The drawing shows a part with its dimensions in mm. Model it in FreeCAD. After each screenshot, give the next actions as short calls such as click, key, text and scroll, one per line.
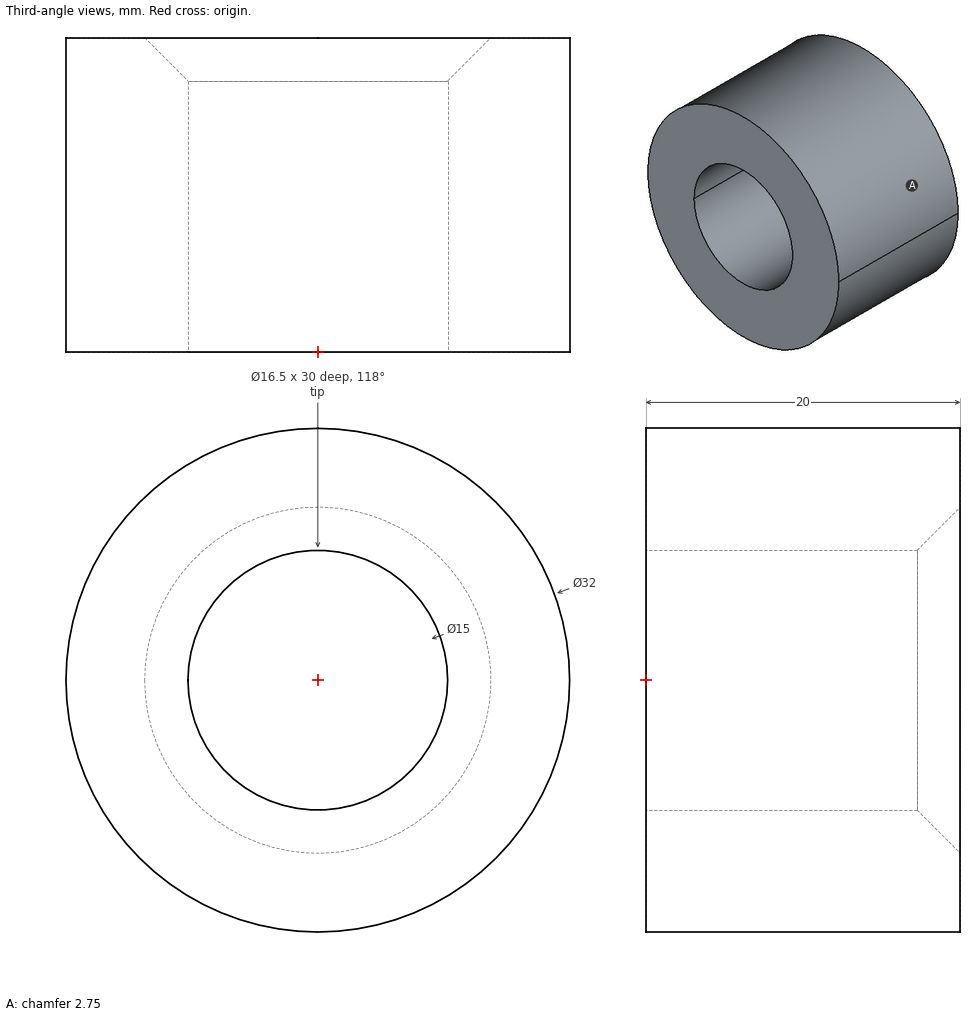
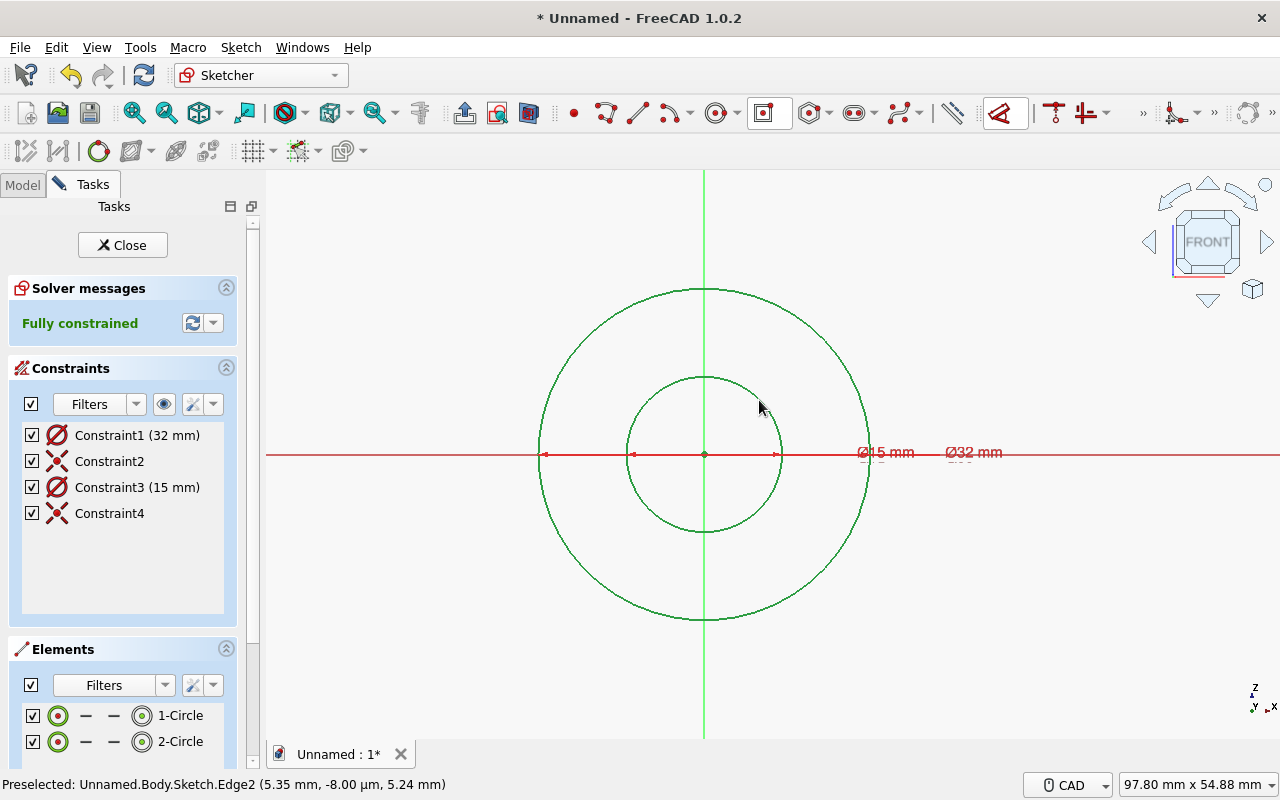
click(123, 245)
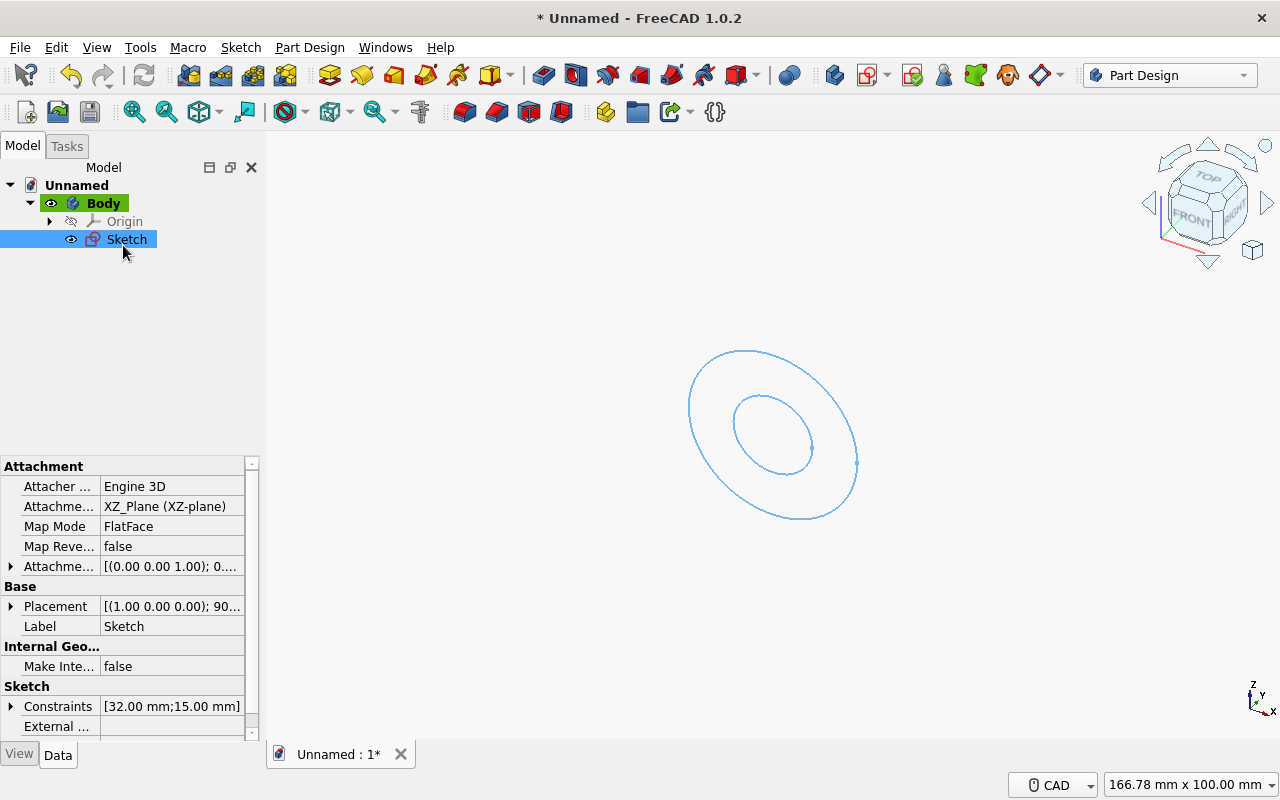
click(330, 76)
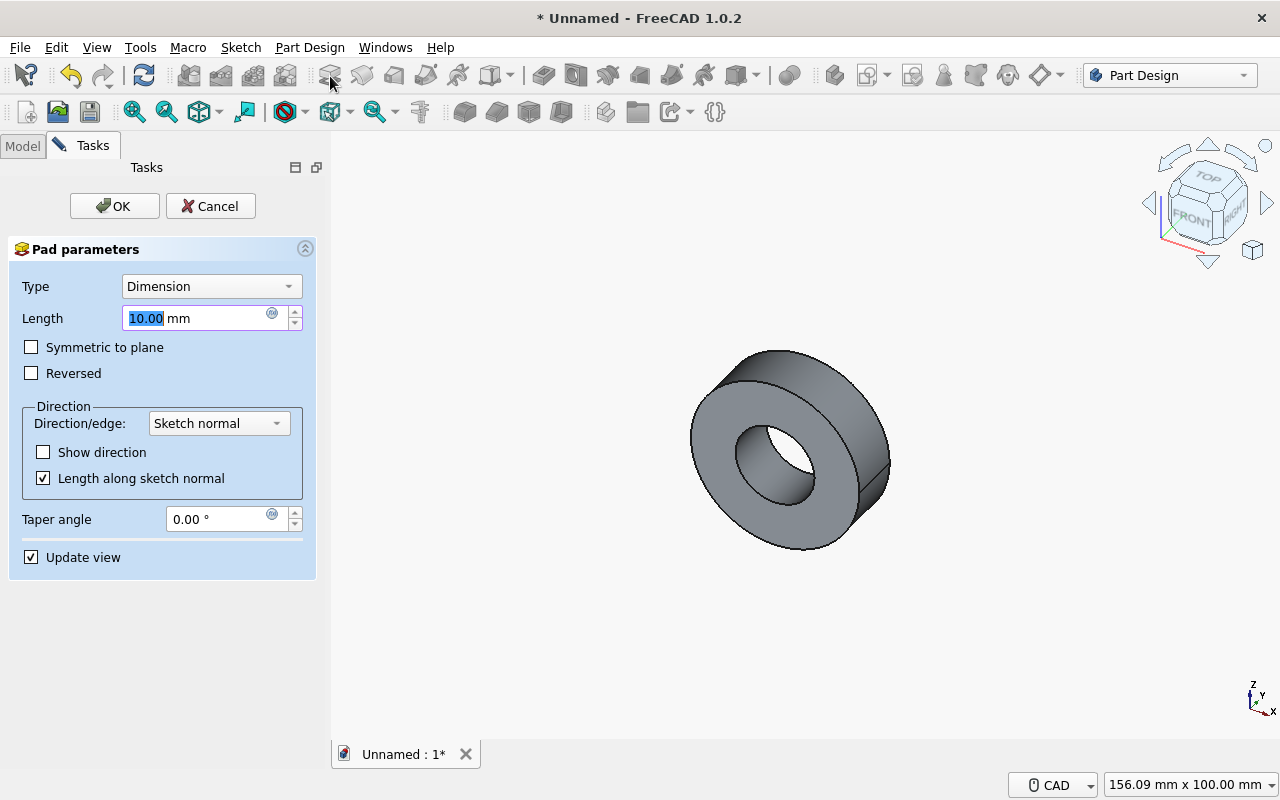
text(20)
key(Tab)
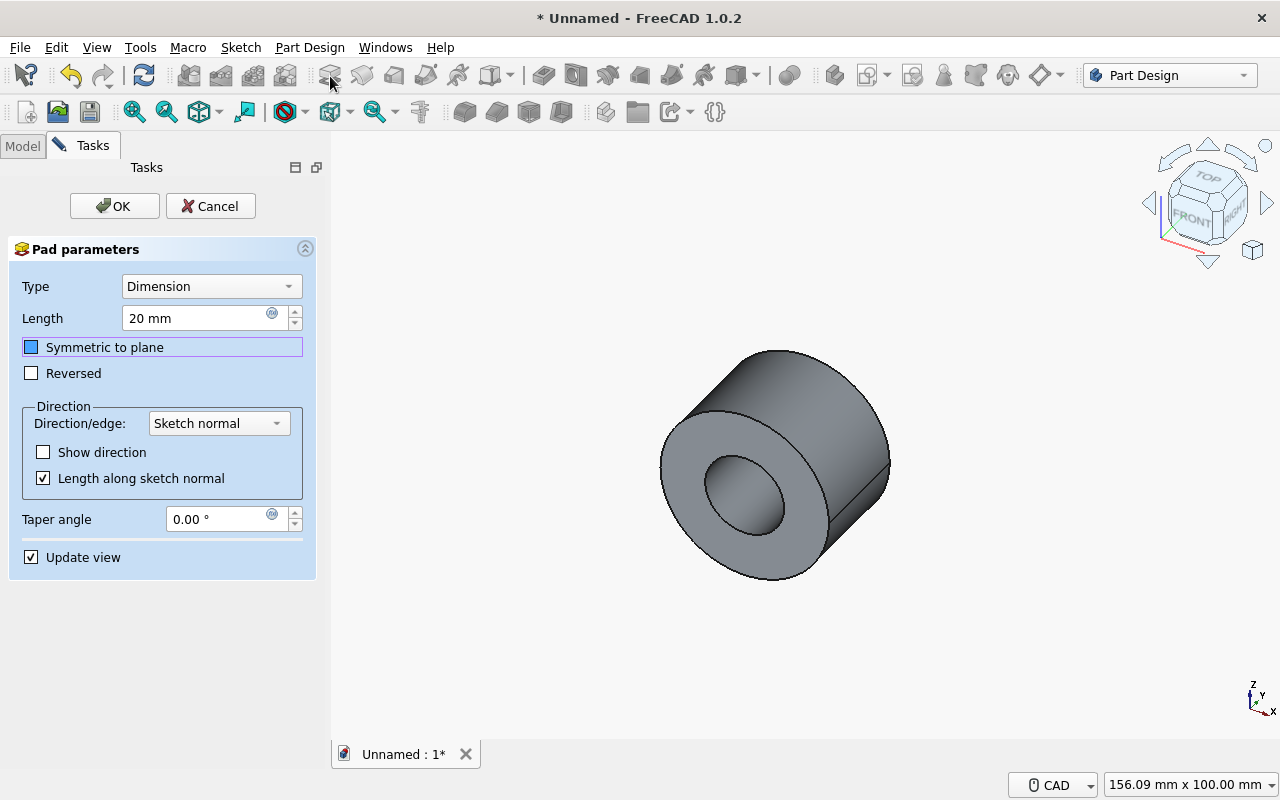
click(30, 373)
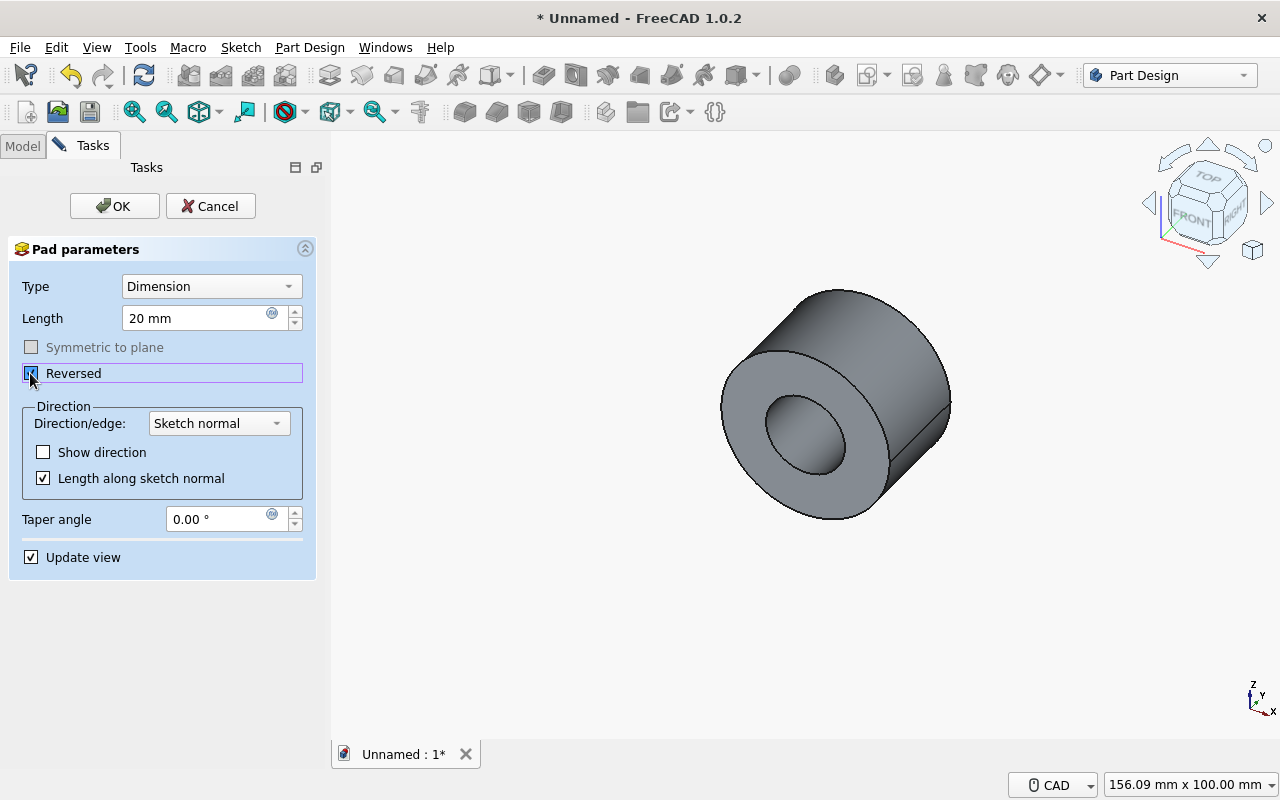
click(115, 206)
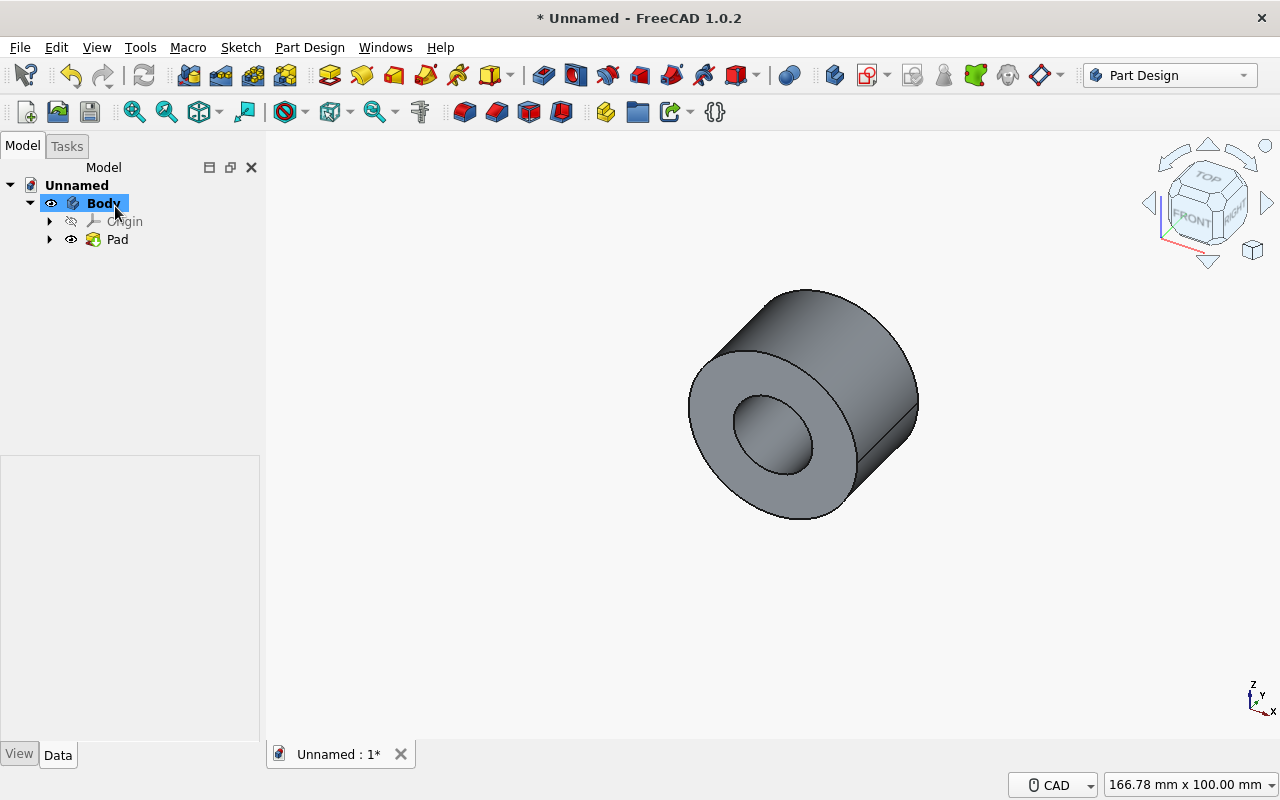
key(4)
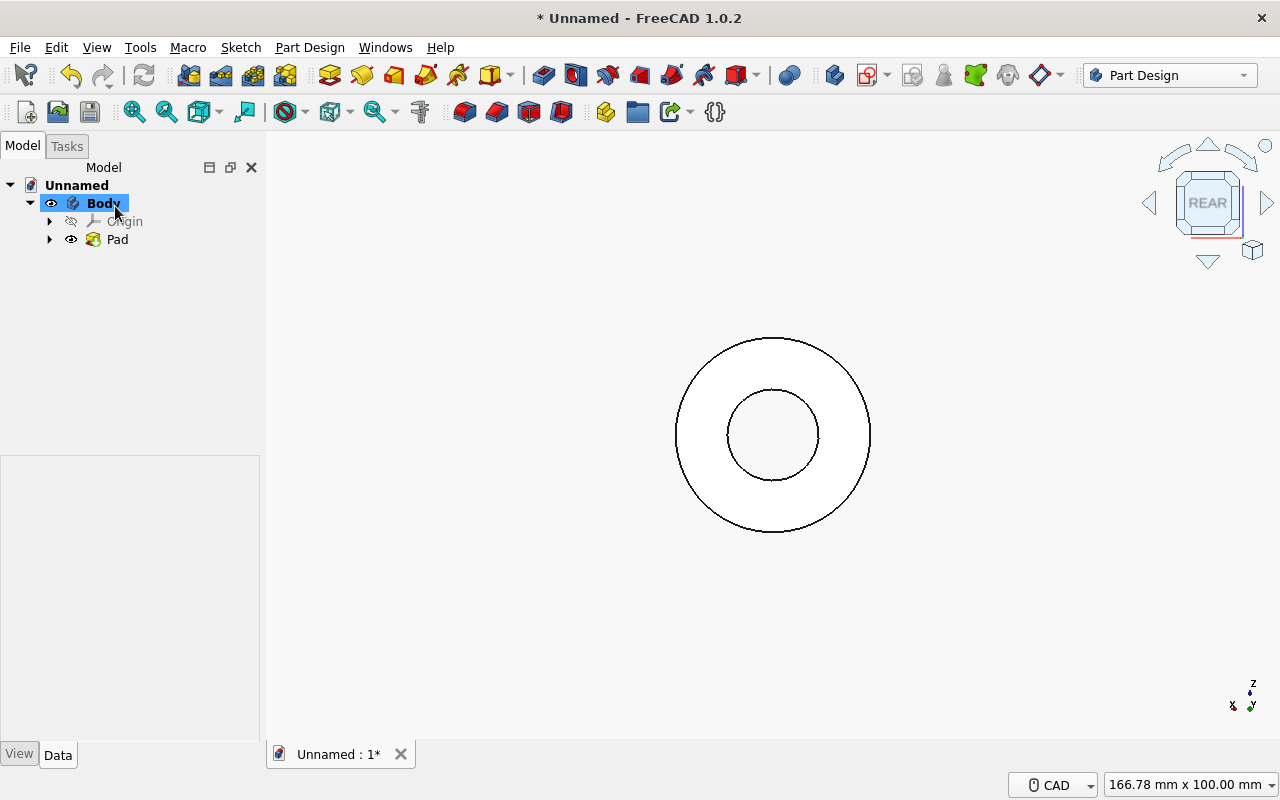
key(v)
key(f)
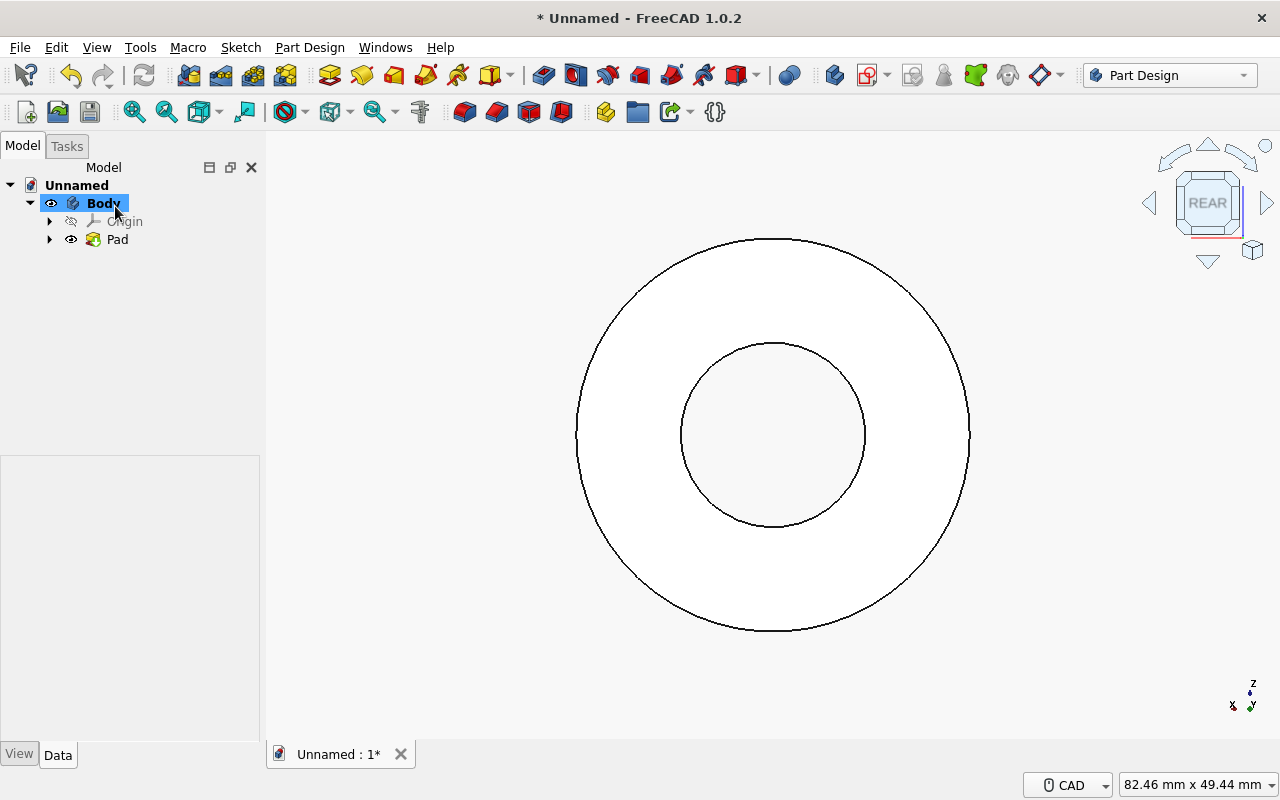
click(885, 546)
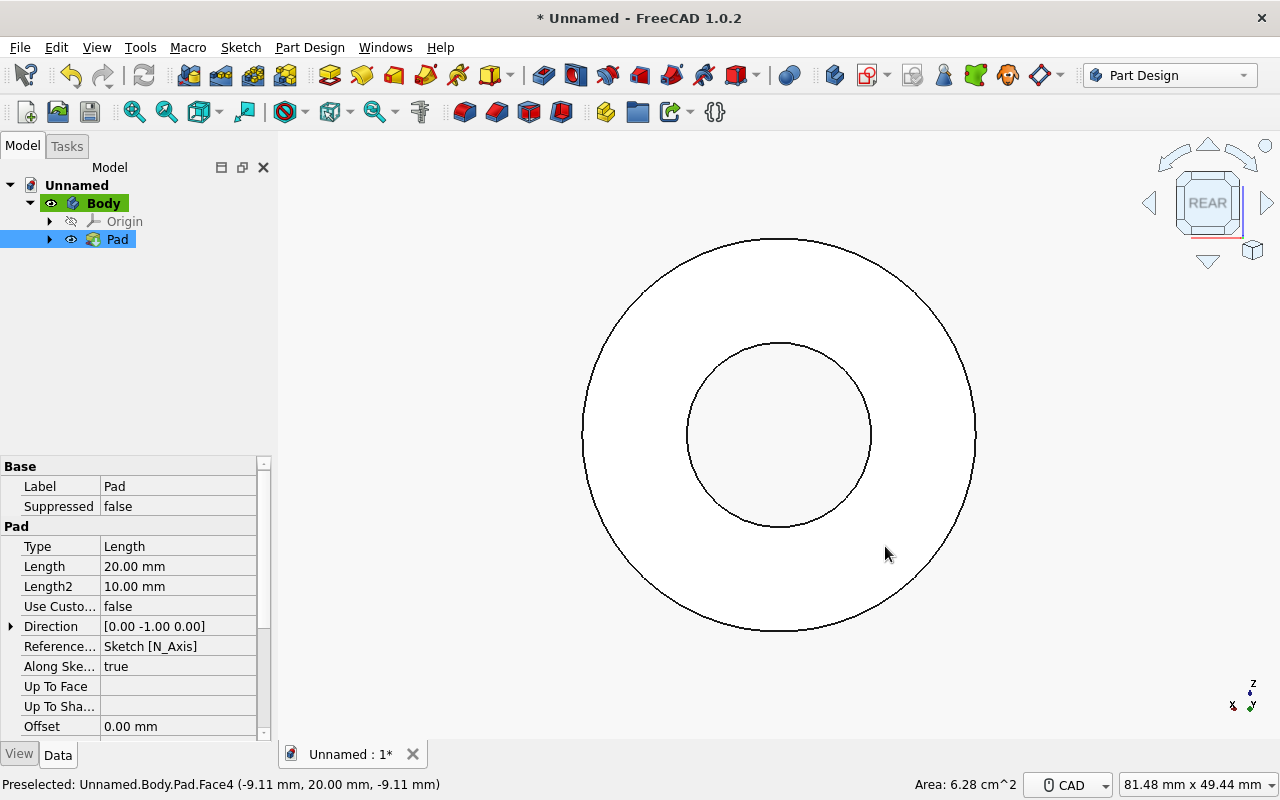
click(868, 76)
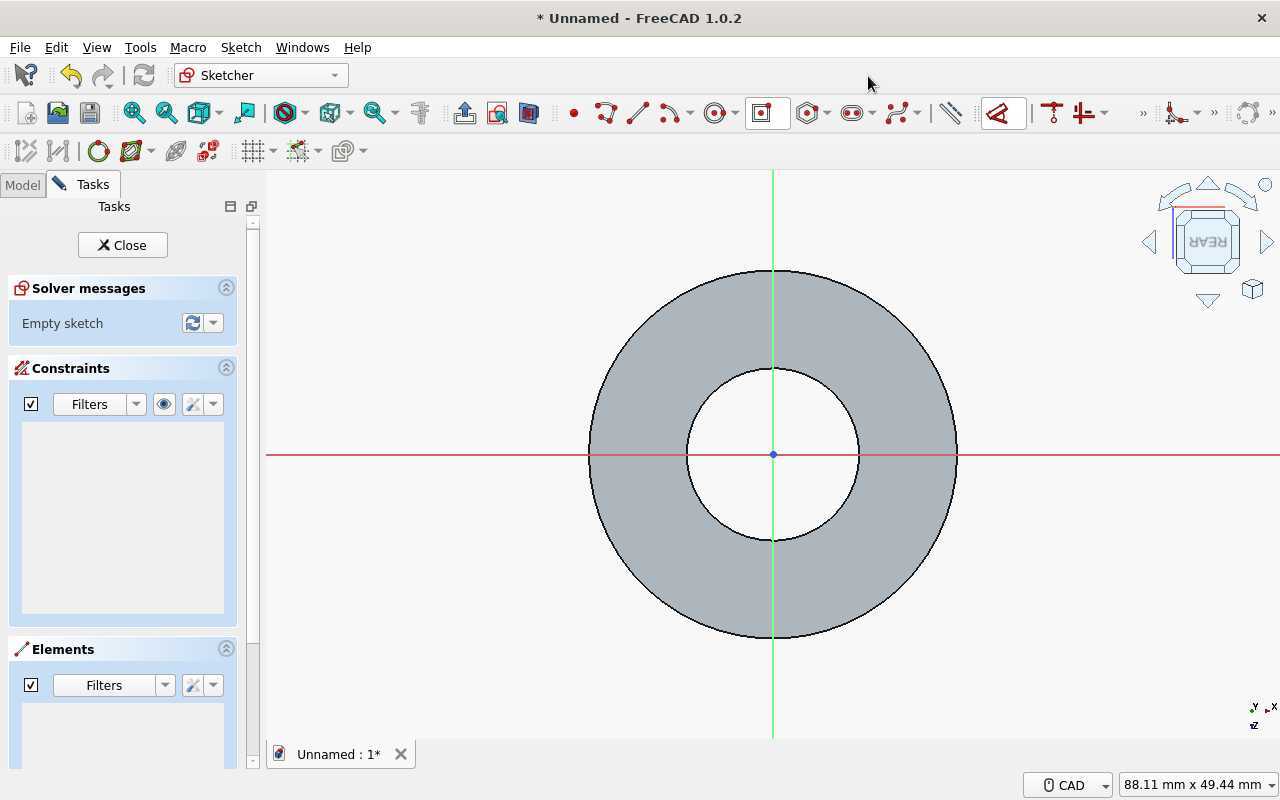
scroll(856, 454, up, 3)